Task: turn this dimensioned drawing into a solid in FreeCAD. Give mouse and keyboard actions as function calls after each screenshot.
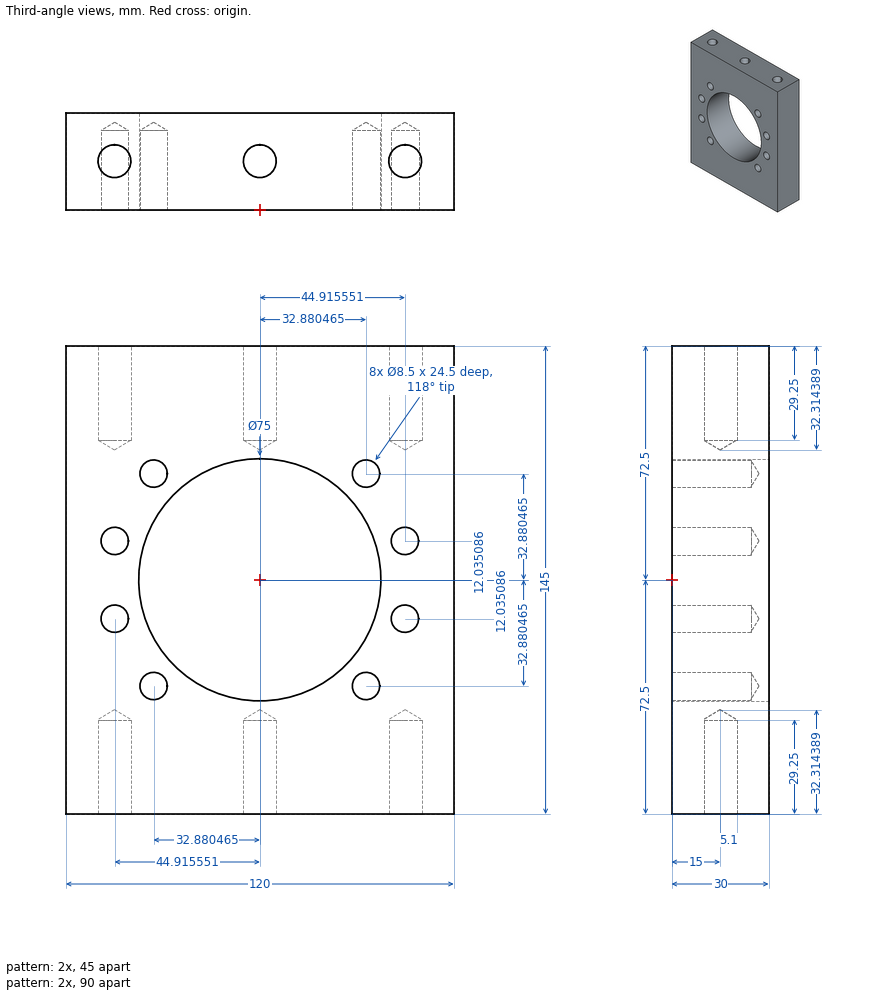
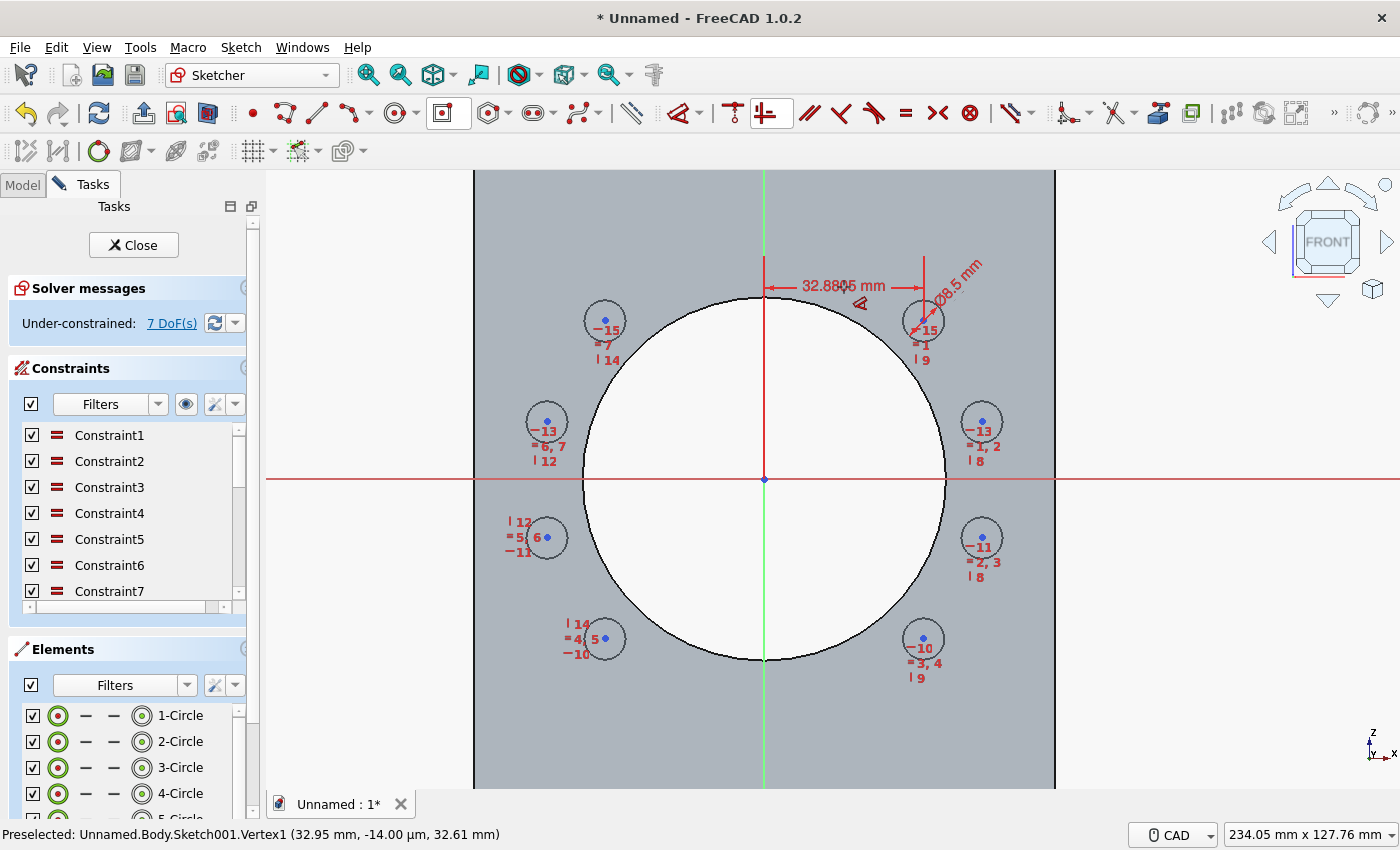
click(924, 321)
click(958, 364)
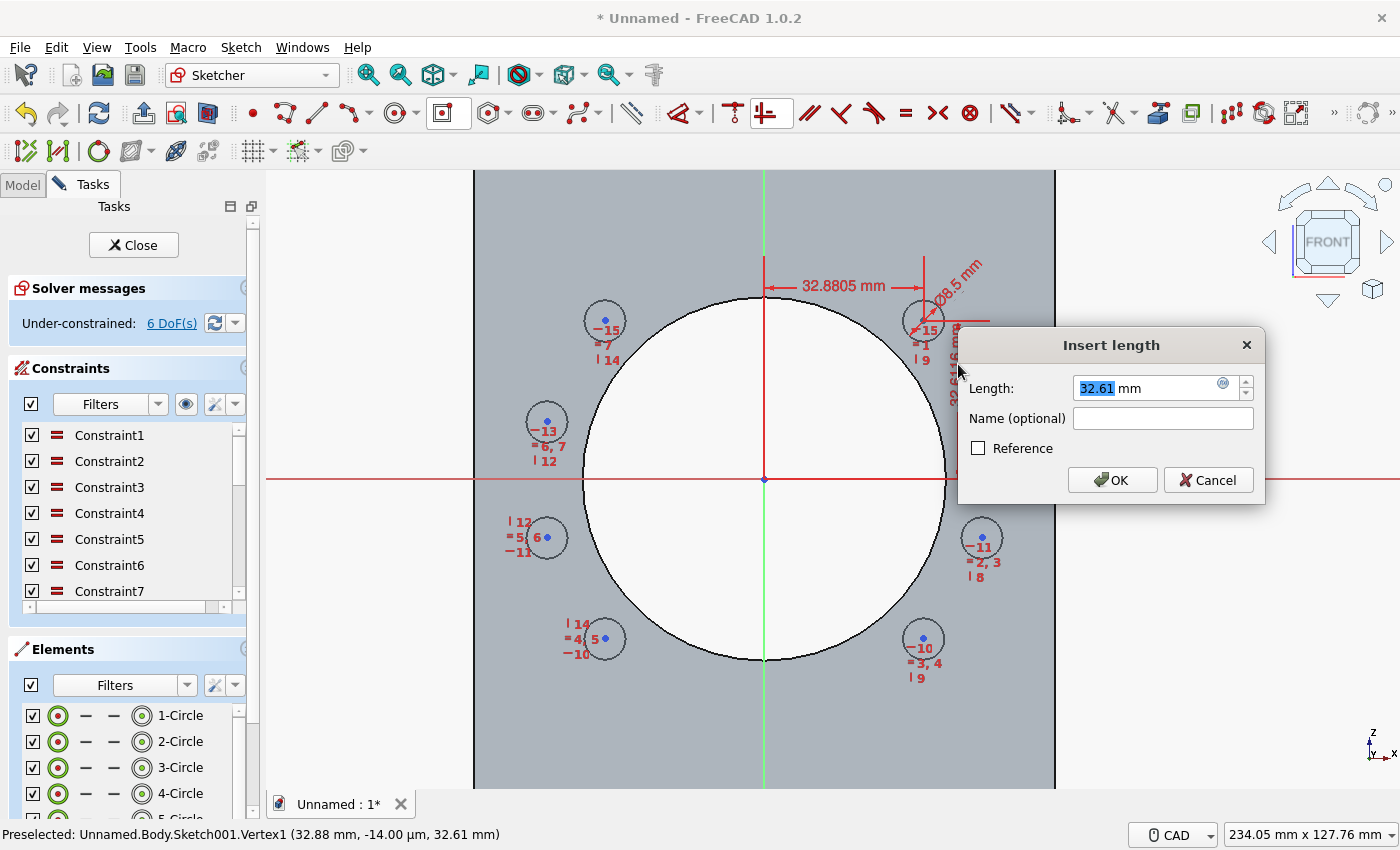
text(32.880465)
key(Return)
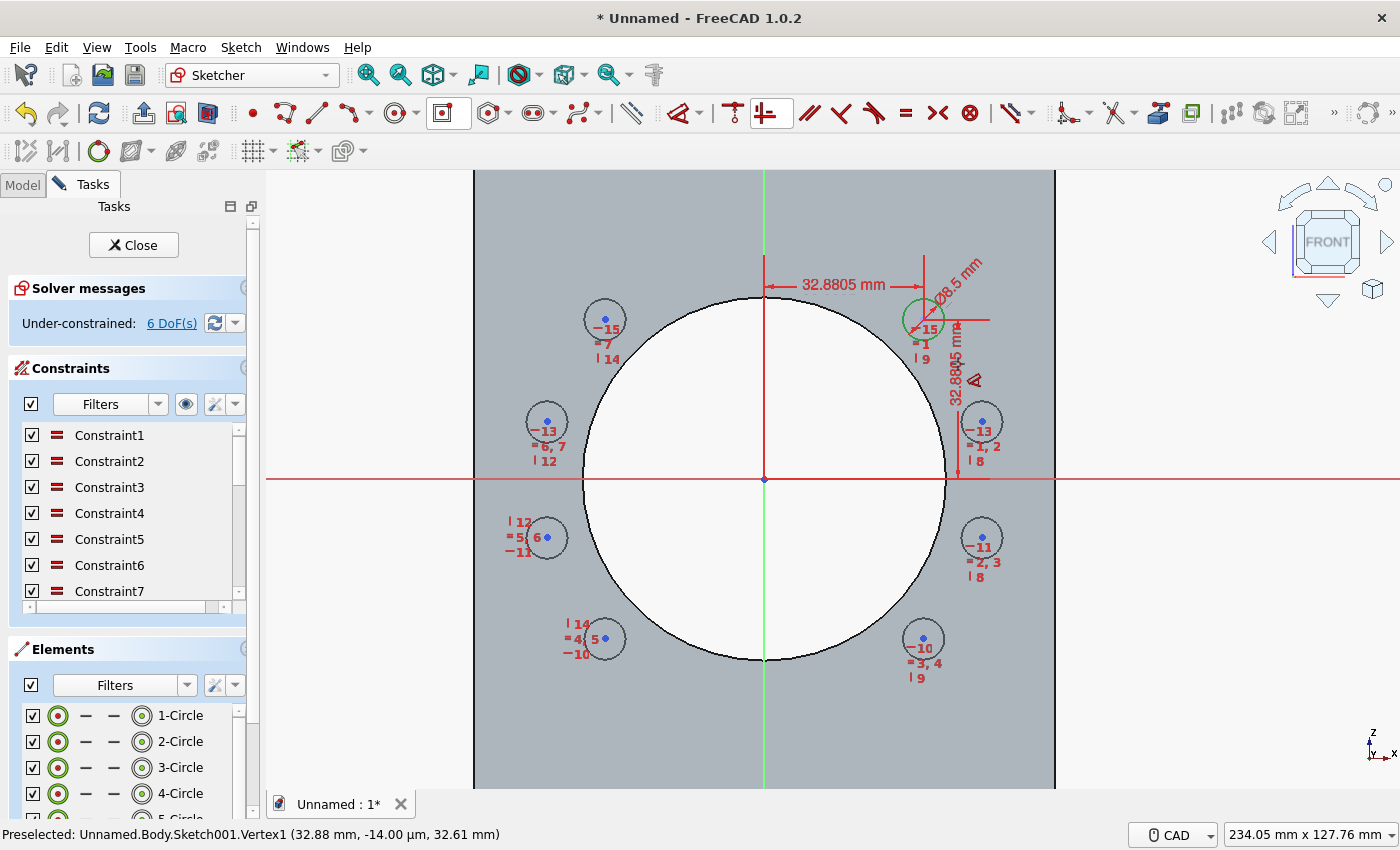
click(982, 422)
click(873, 388)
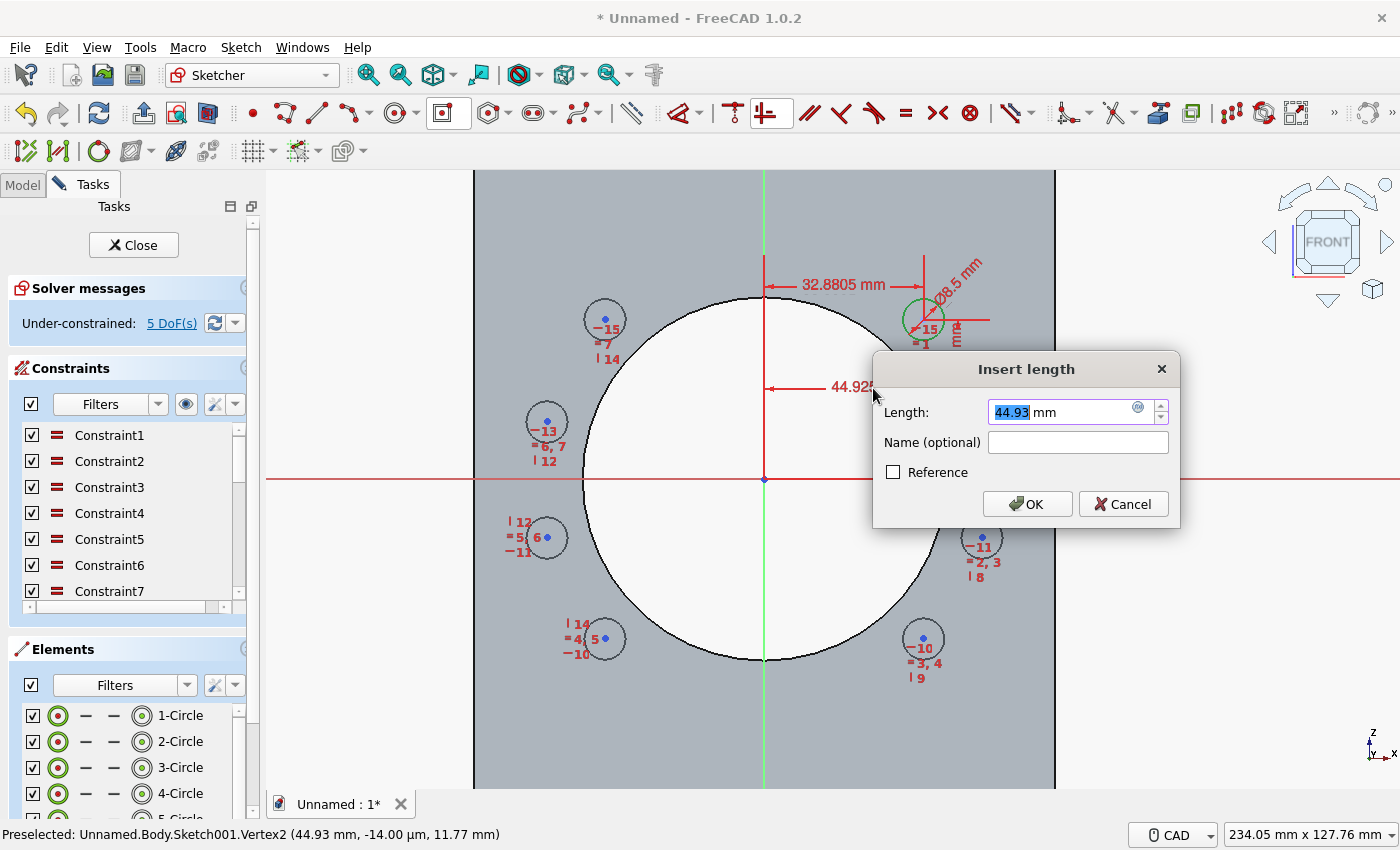
text(44.915551)
key(Return)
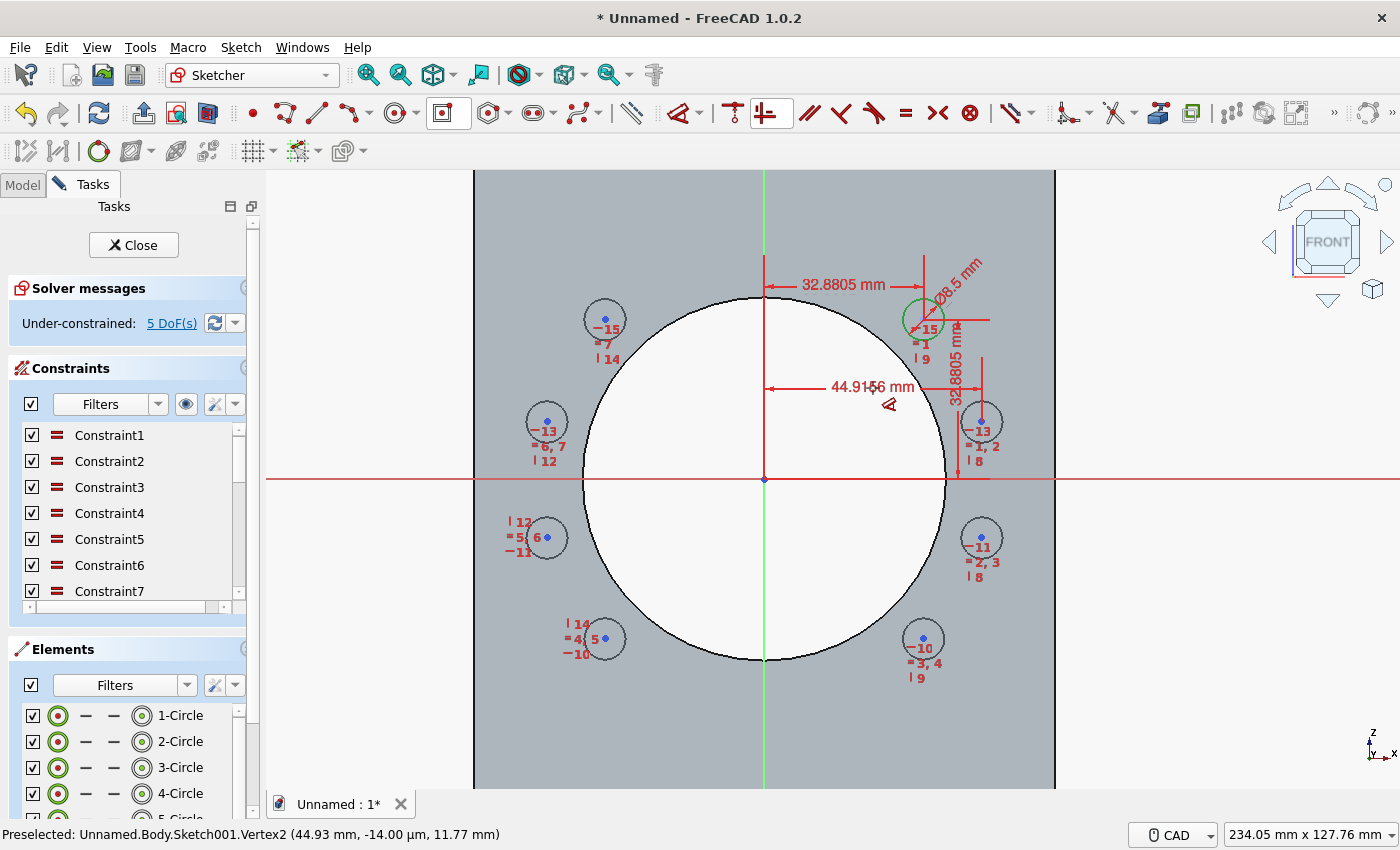
click(982, 422)
click(1016, 451)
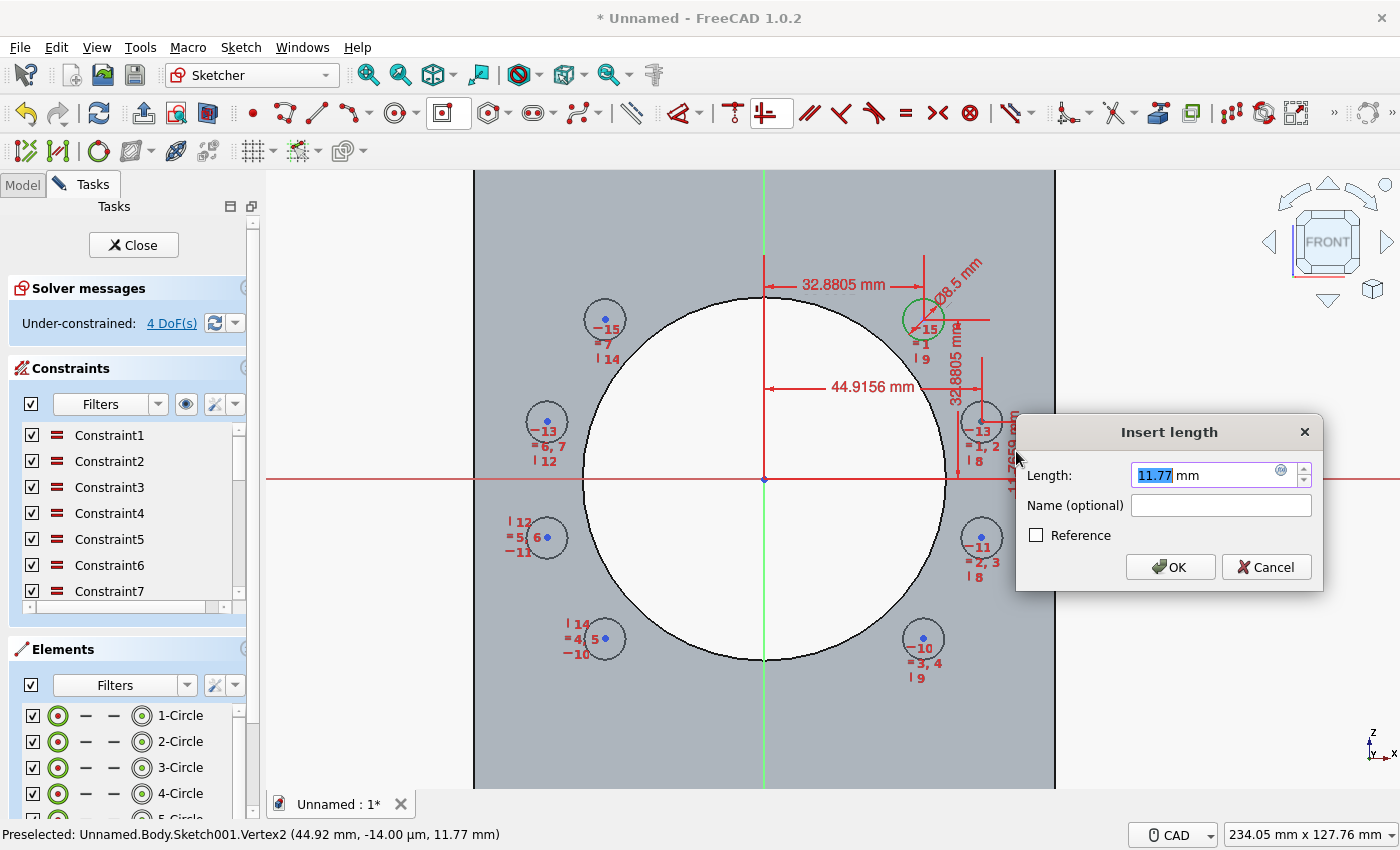
text(12.035086)
key(Return)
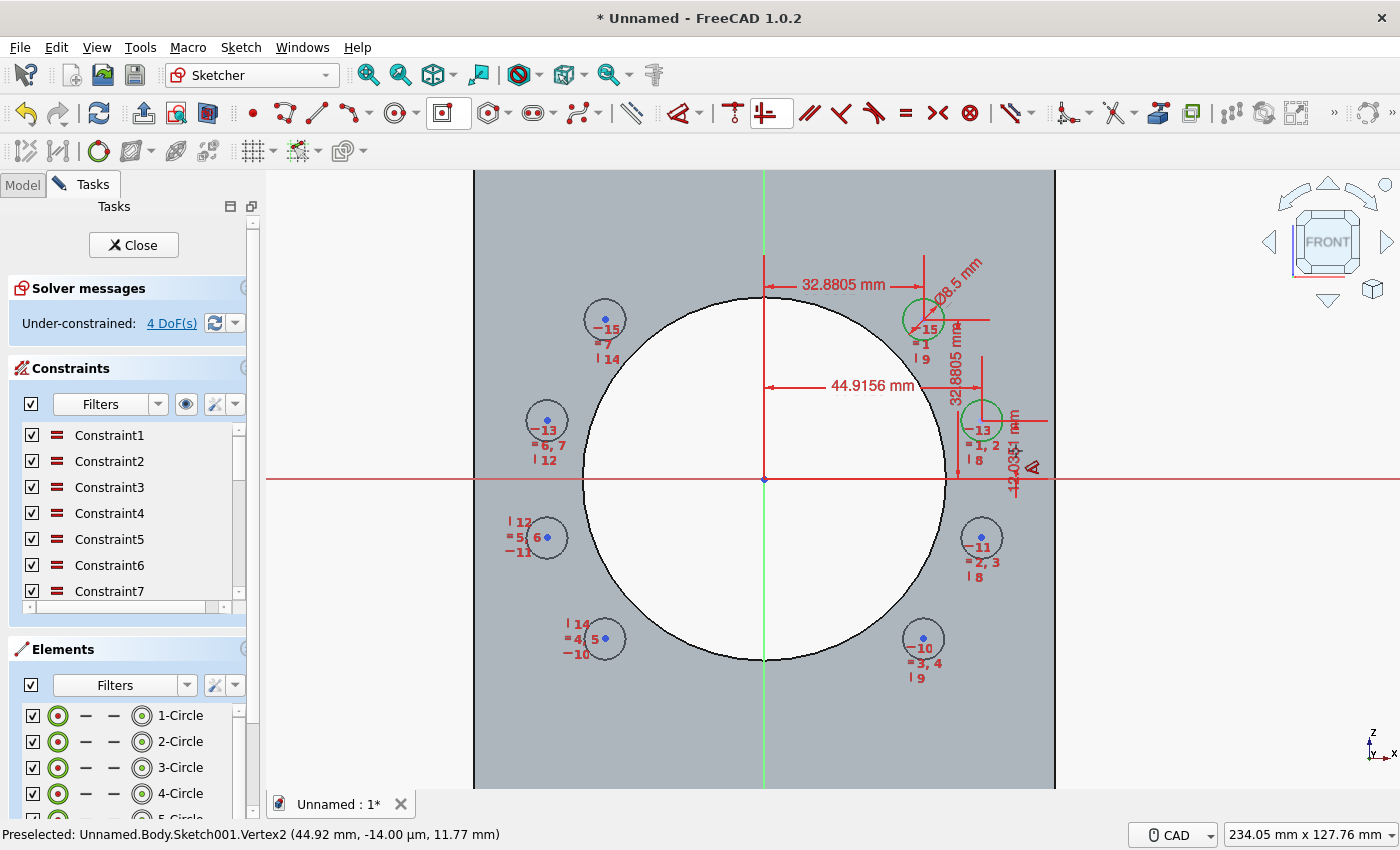
click(982, 538)
click(1016, 509)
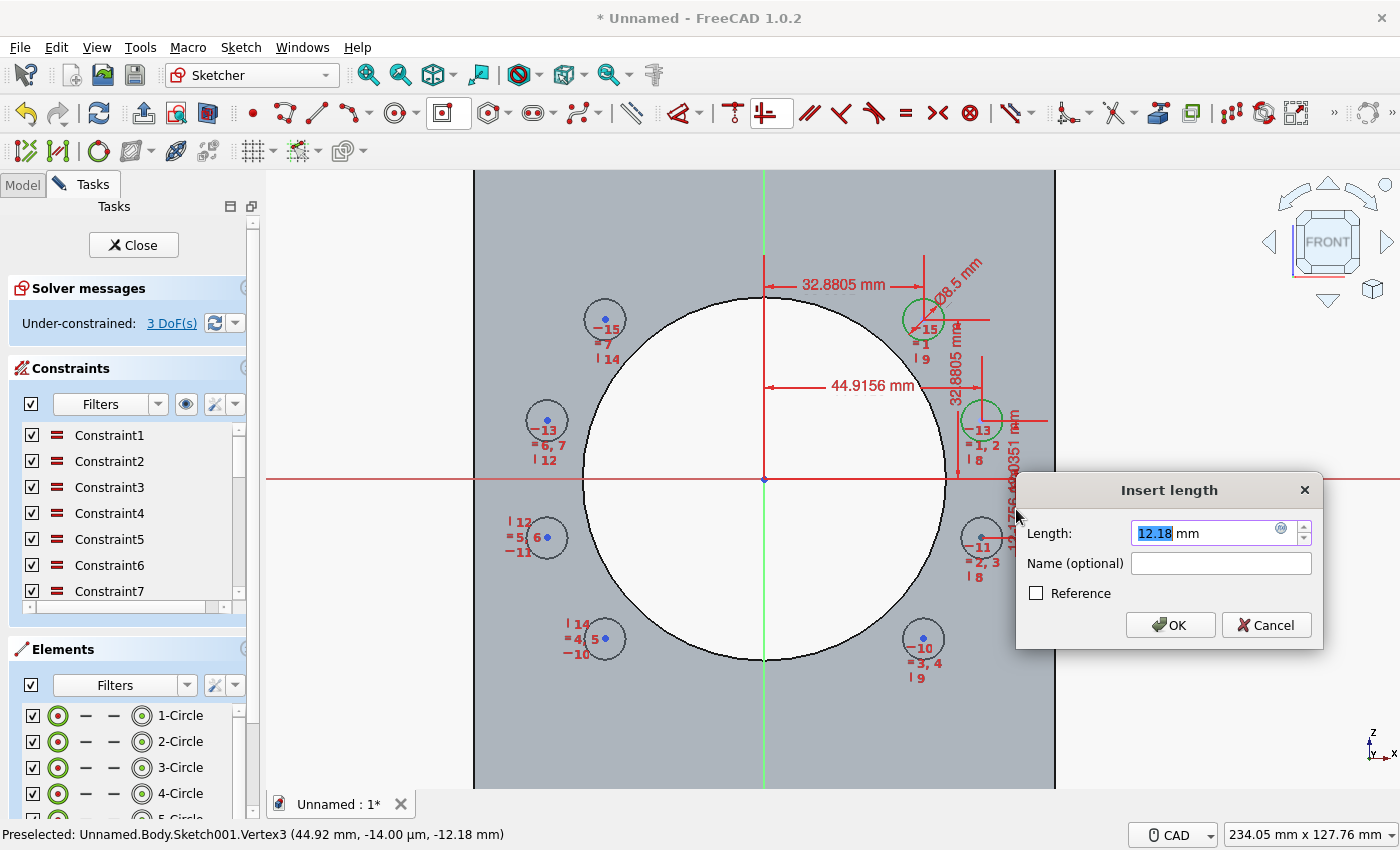
text(12.035086)
key(Return)